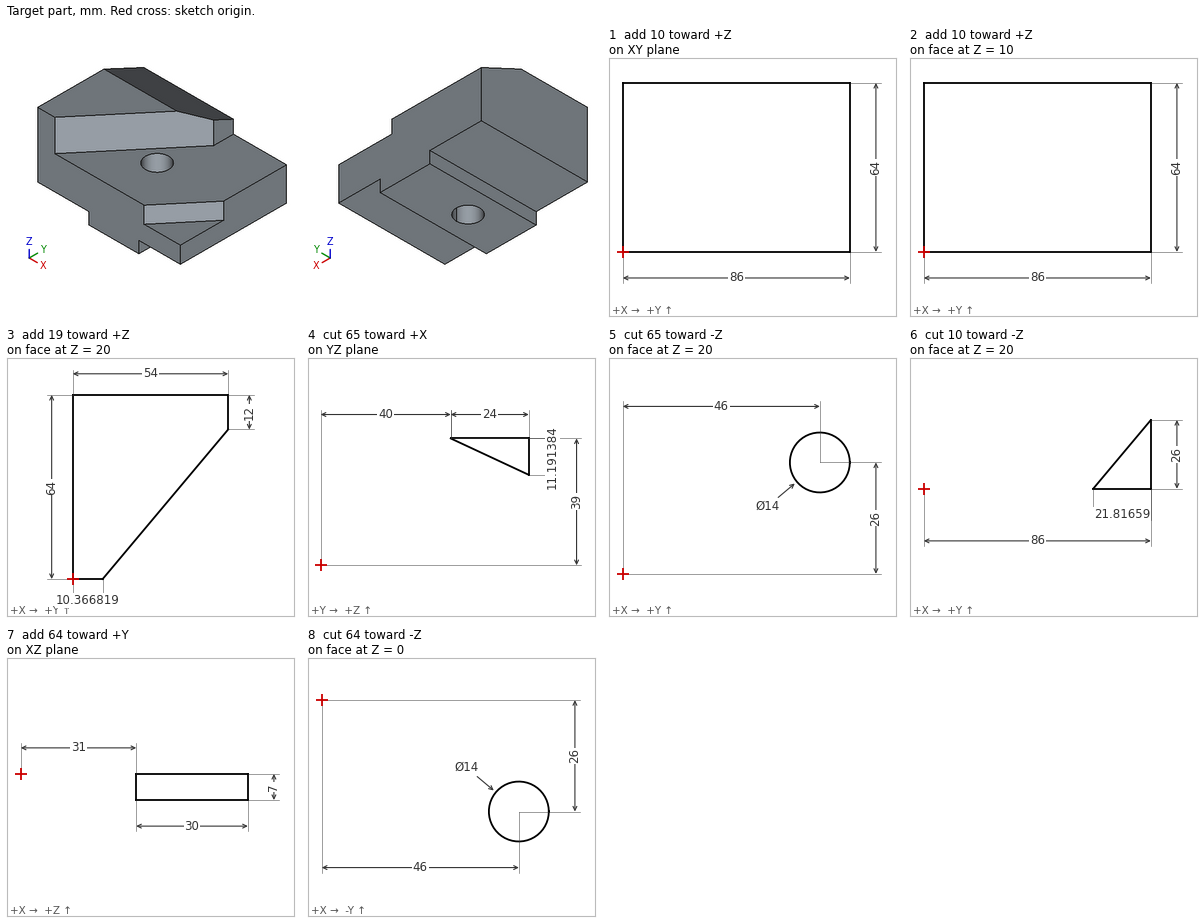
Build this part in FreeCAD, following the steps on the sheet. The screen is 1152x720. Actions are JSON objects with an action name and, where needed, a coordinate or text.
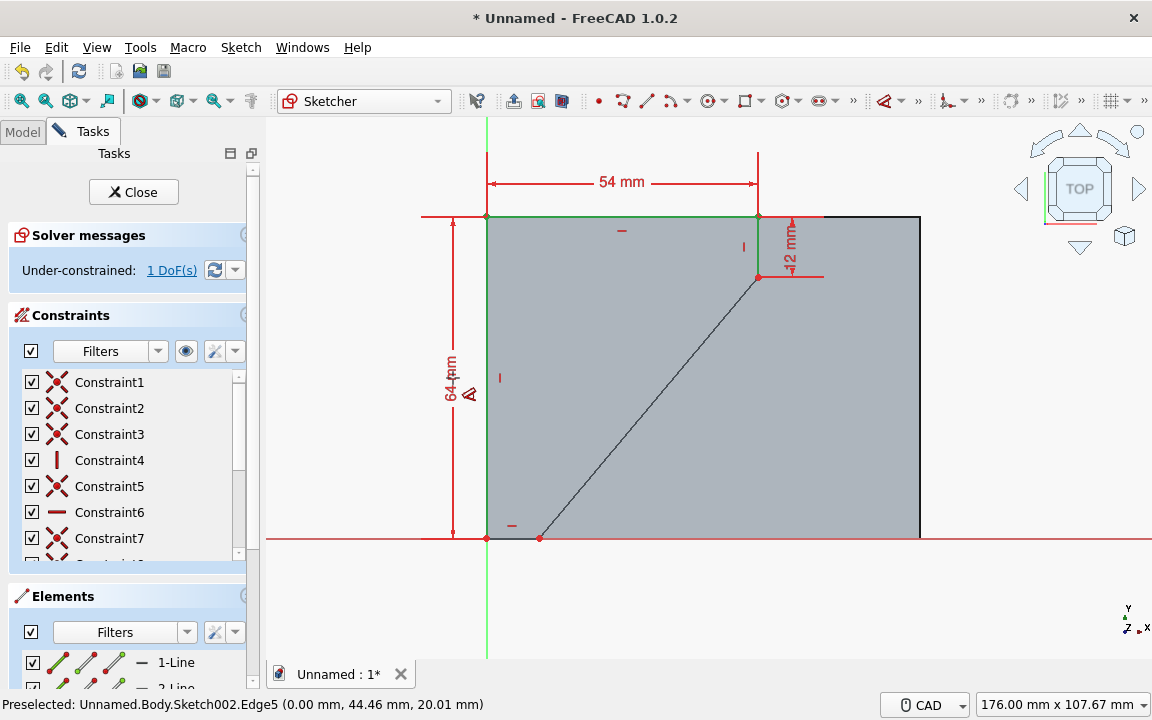
{"action": "left_click", "coordinate": [502, 539]}
{"action": "left_click", "coordinate": [513, 573]}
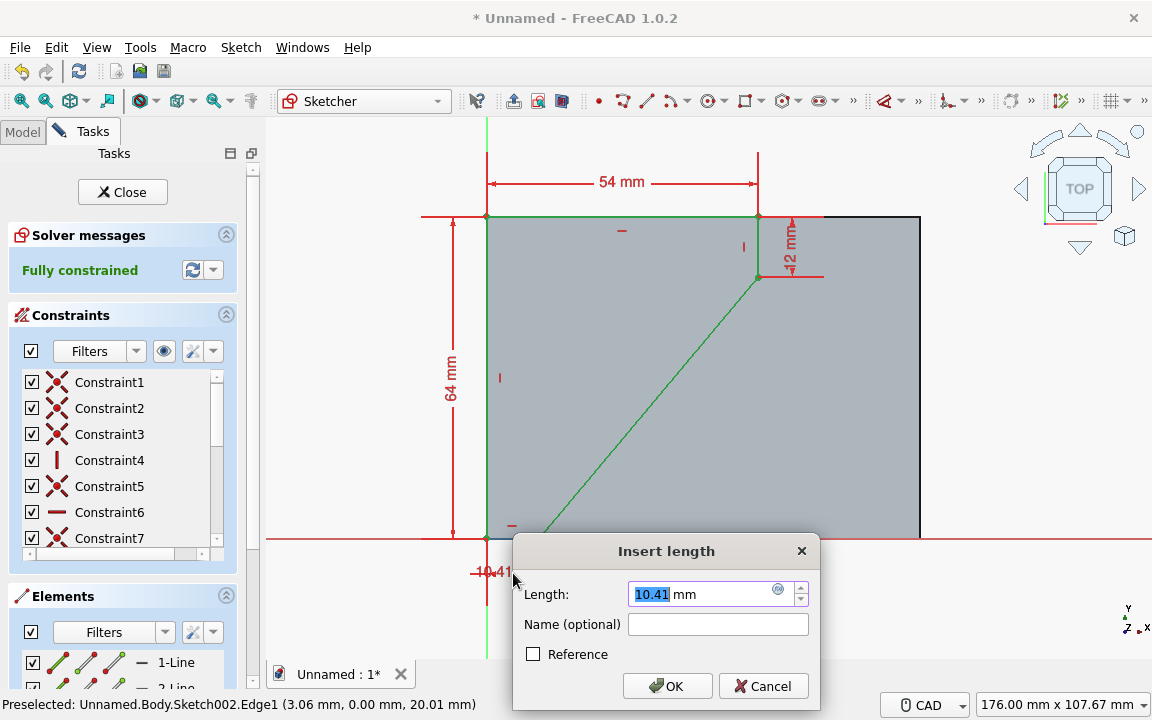
{"action": "type", "text": "10.366819"}
{"action": "key", "text": "Return"}
{"action": "key", "text": "Escape"}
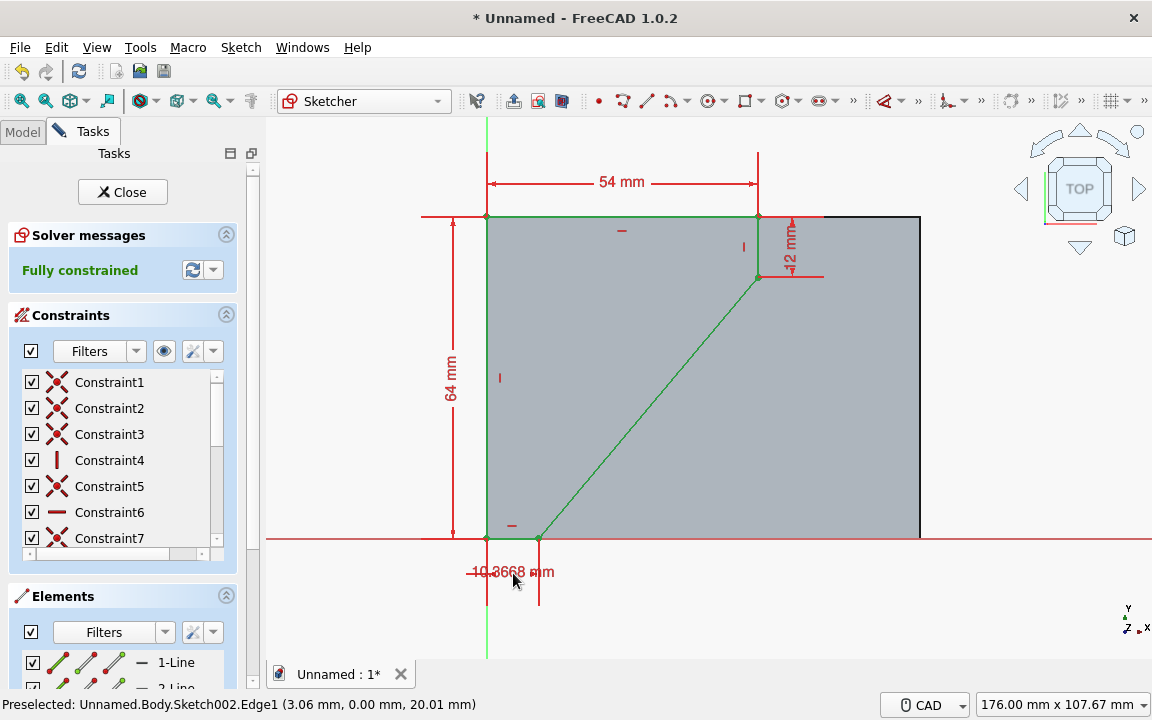
{"action": "left_click", "coordinate": [123, 192]}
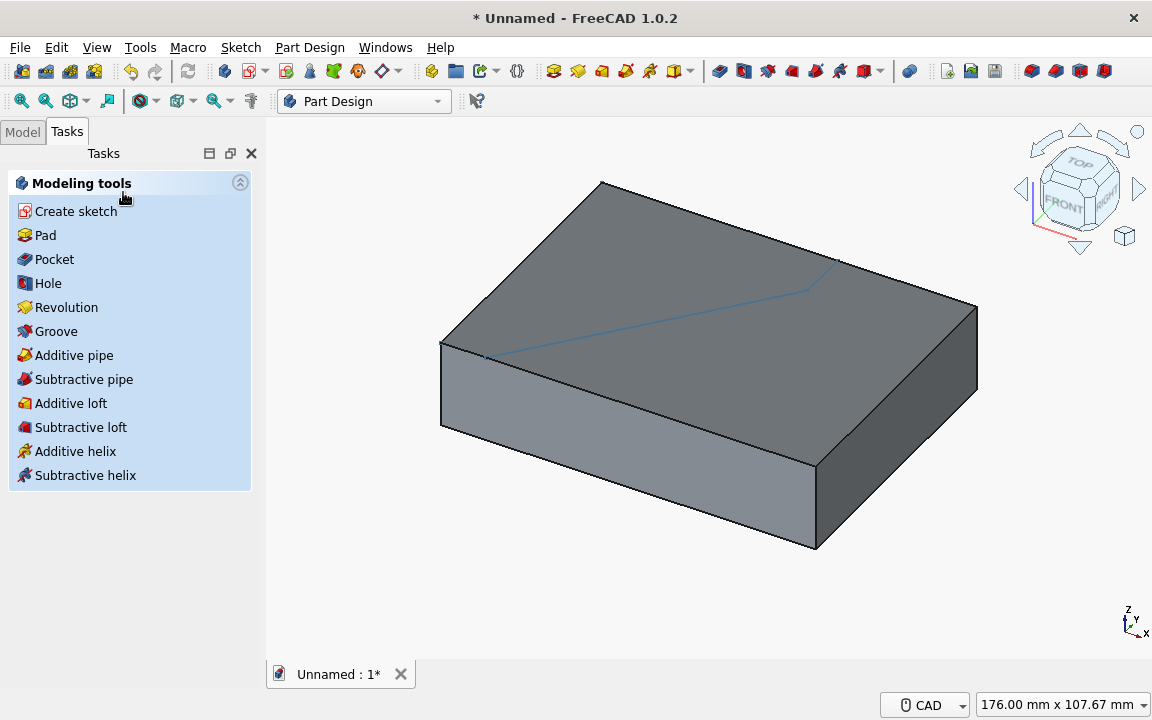
{"action": "left_click", "coordinate": [554, 72]}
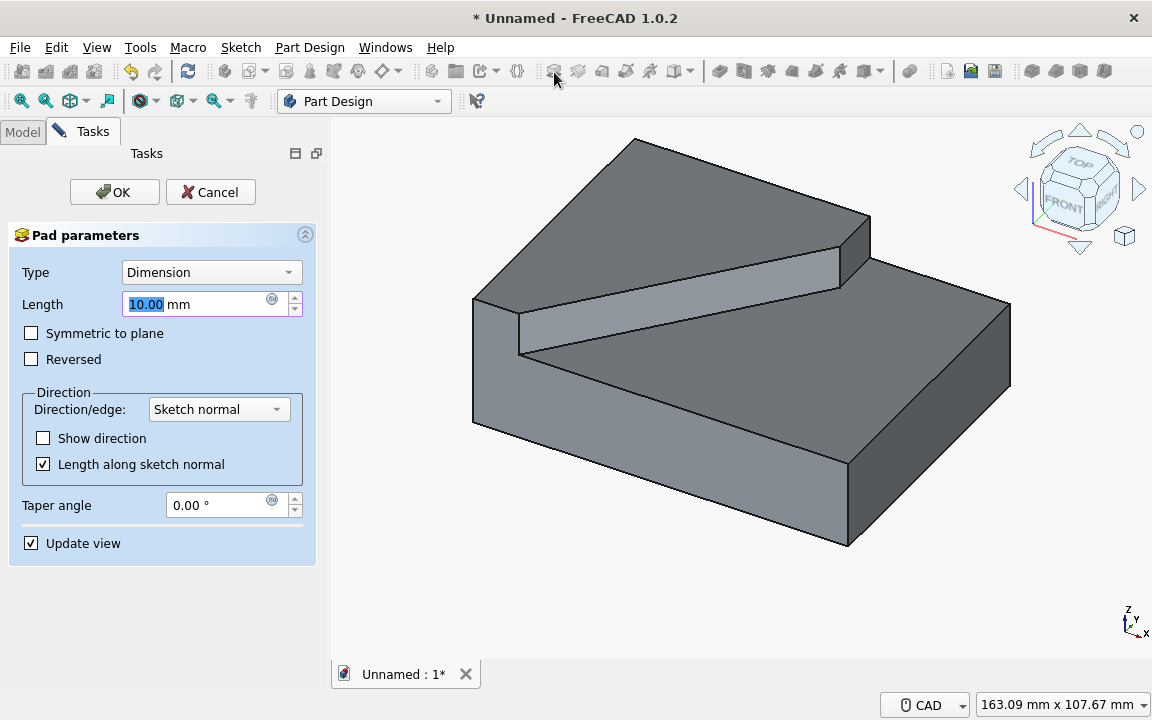
{"action": "type", "text": "19"}
{"action": "key", "text": "Tab"}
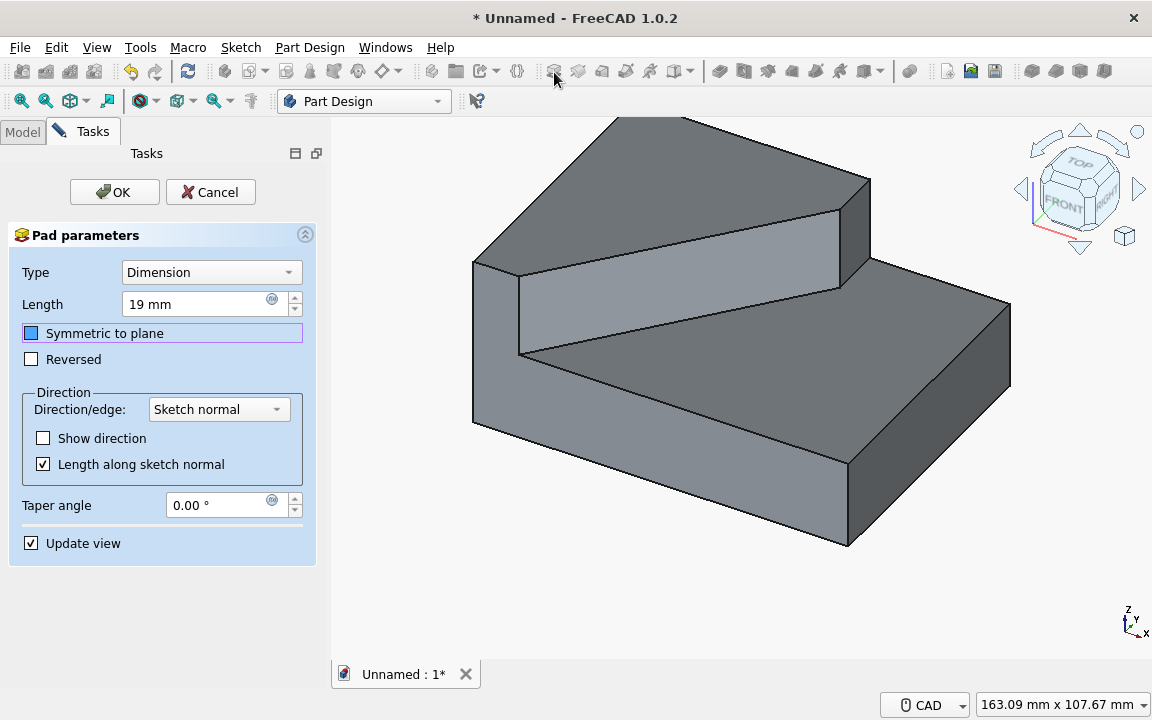
{"action": "left_click", "coordinate": [115, 192]}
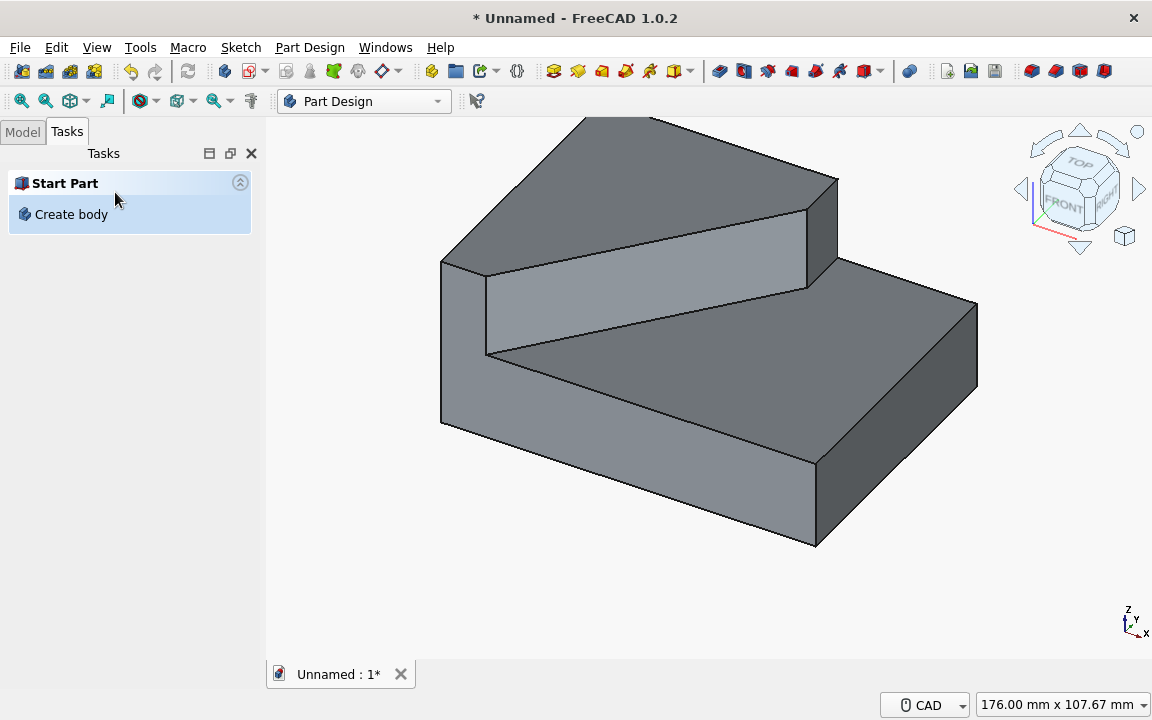
{"action": "left_click", "coordinate": [22, 102]}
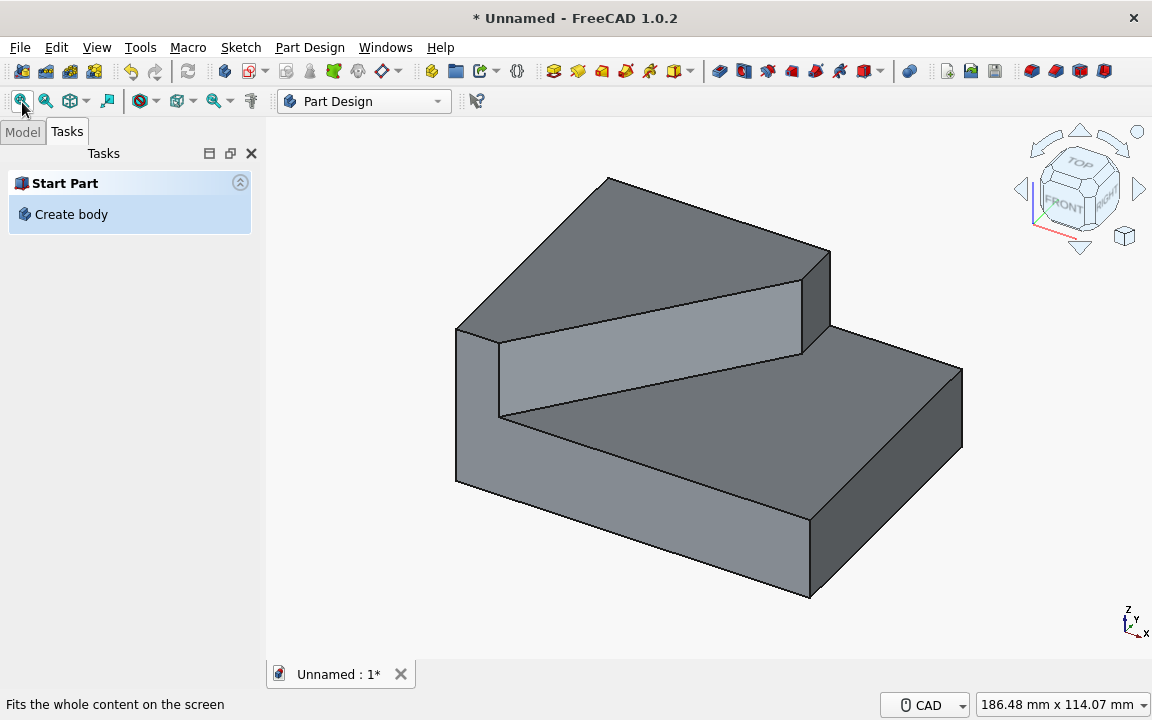
{"action": "left_click", "coordinate": [250, 72]}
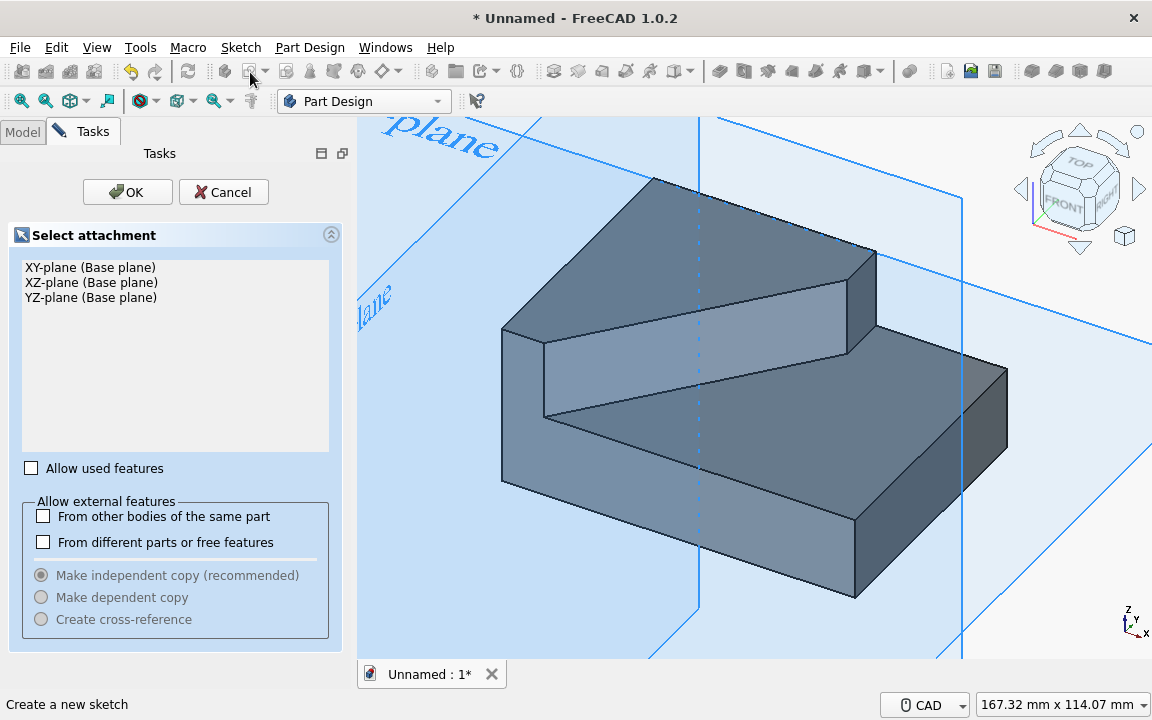
{"action": "left_click", "coordinate": [82, 298]}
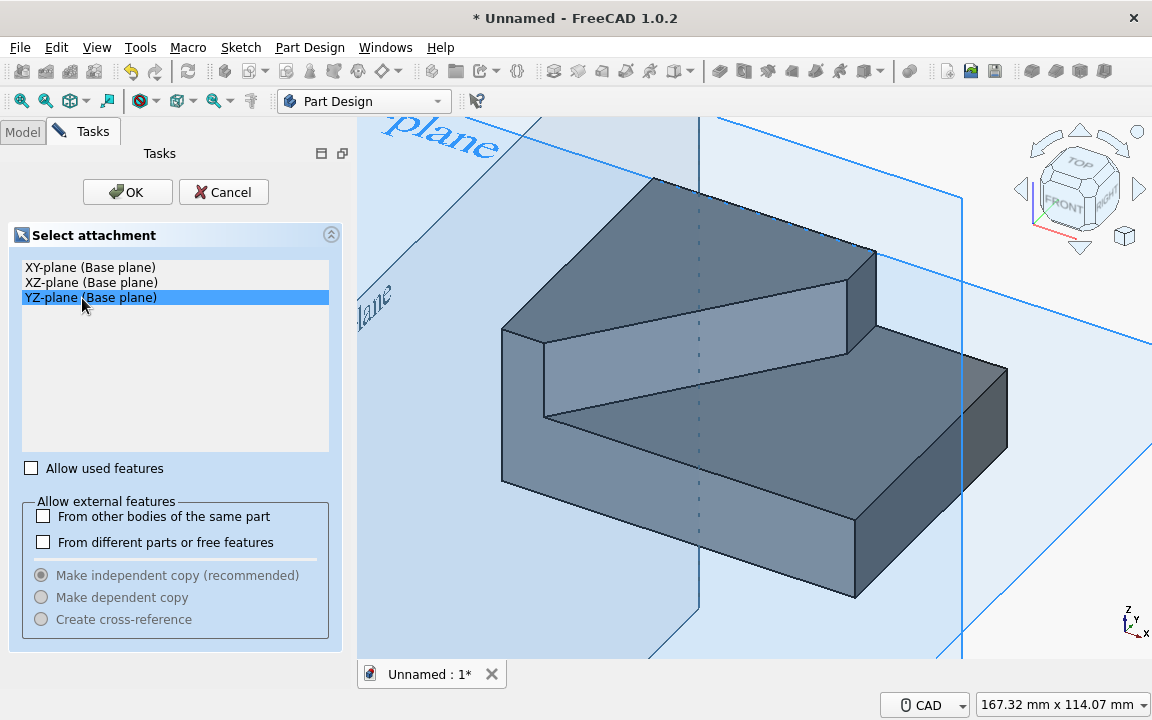
{"action": "left_click", "coordinate": [128, 192]}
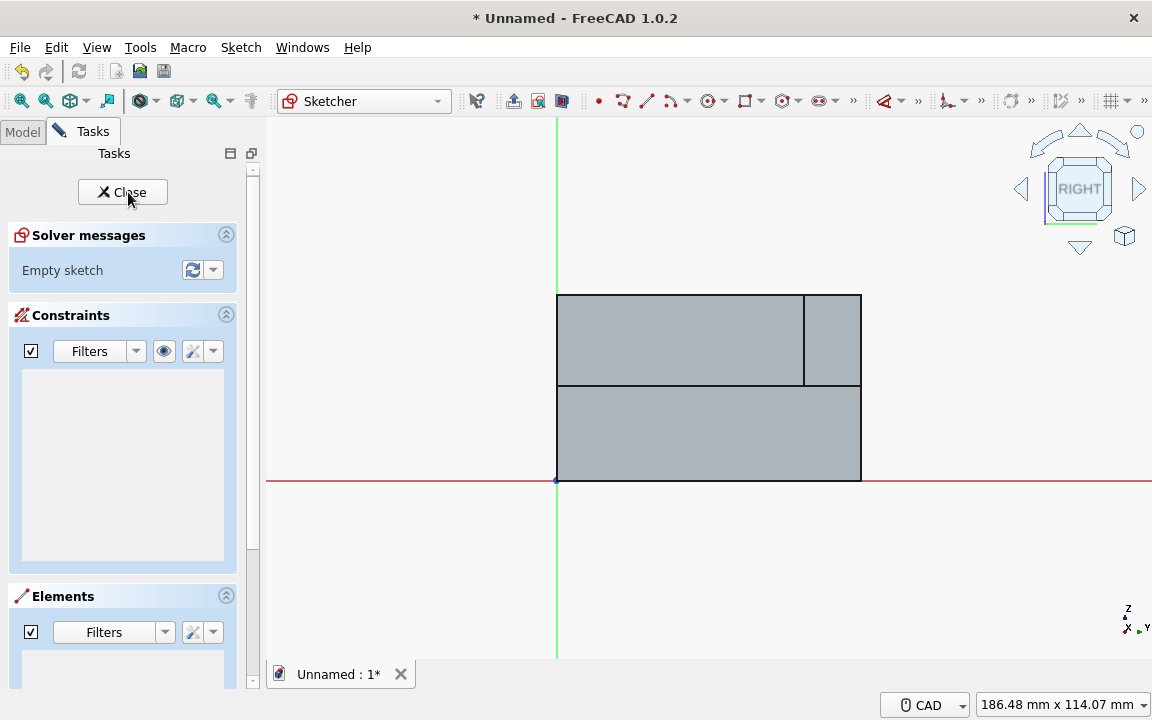
{"action": "left_click", "coordinate": [562, 102]}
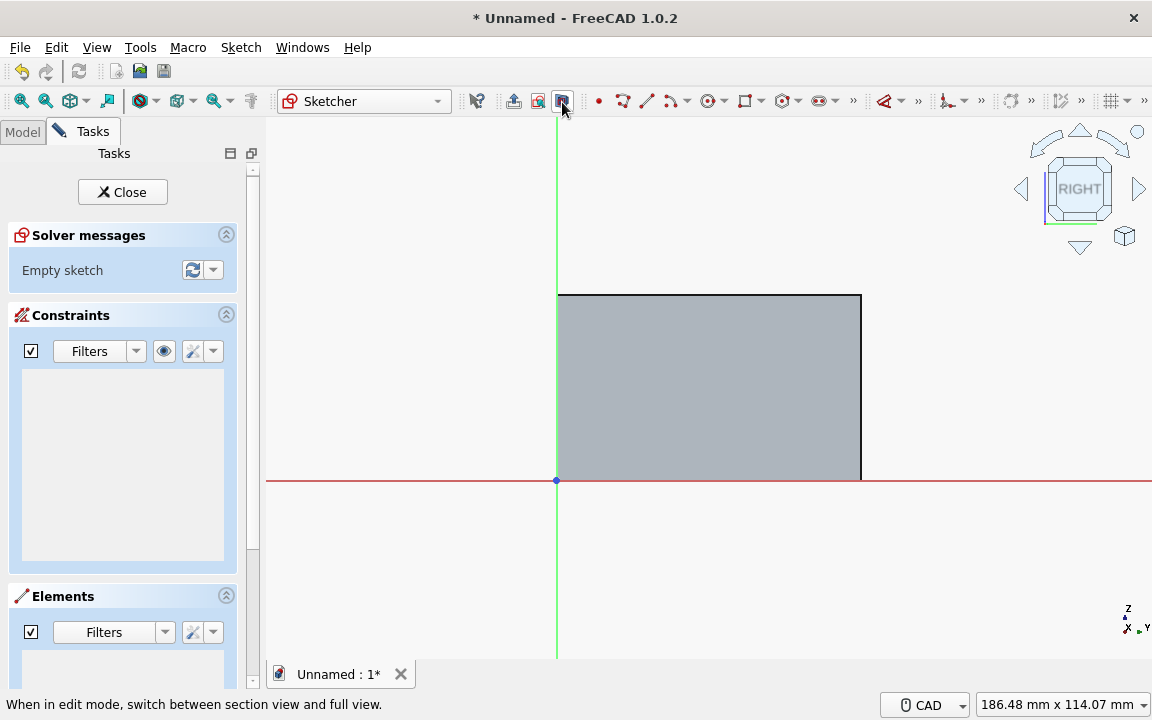
{"action": "scroll", "coordinate": [858, 300], "scroll_direction": "up", "scroll_amount": 7}